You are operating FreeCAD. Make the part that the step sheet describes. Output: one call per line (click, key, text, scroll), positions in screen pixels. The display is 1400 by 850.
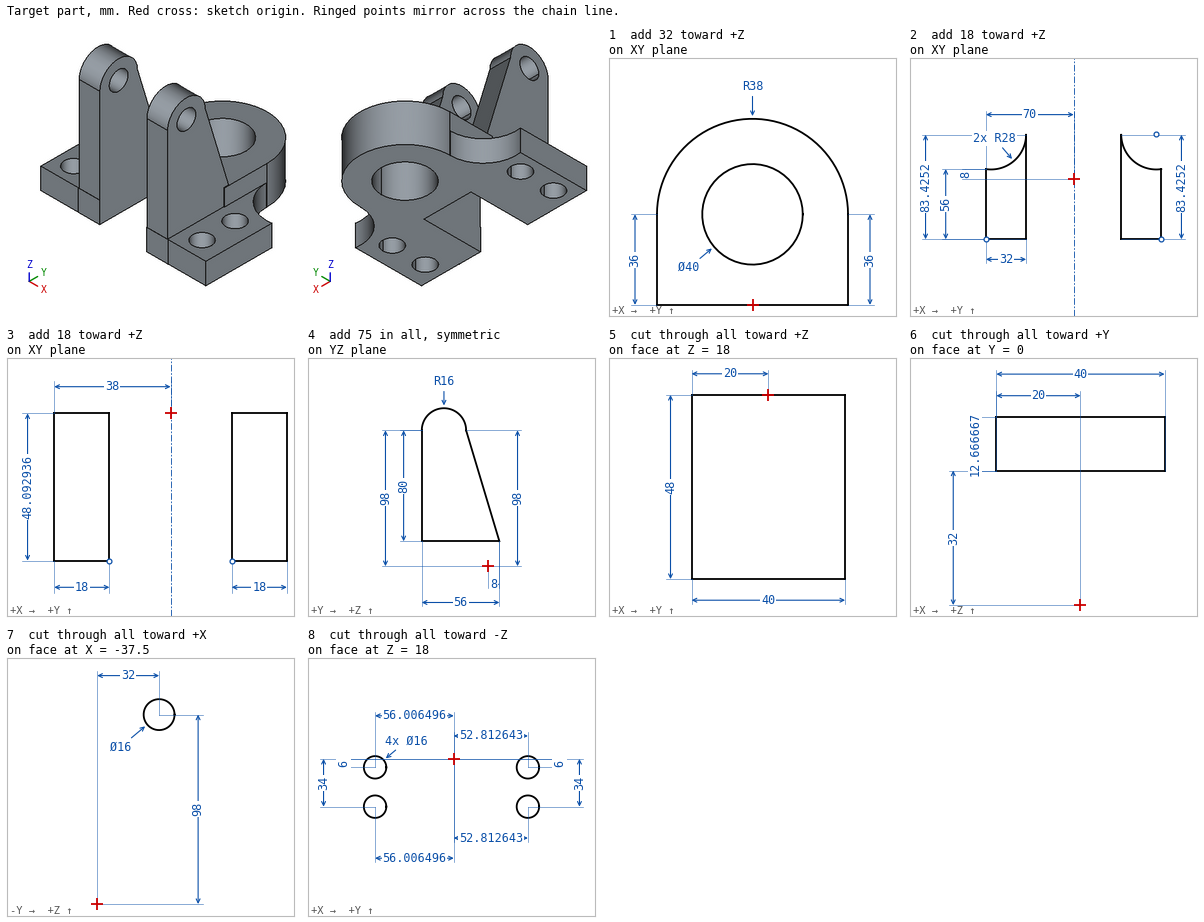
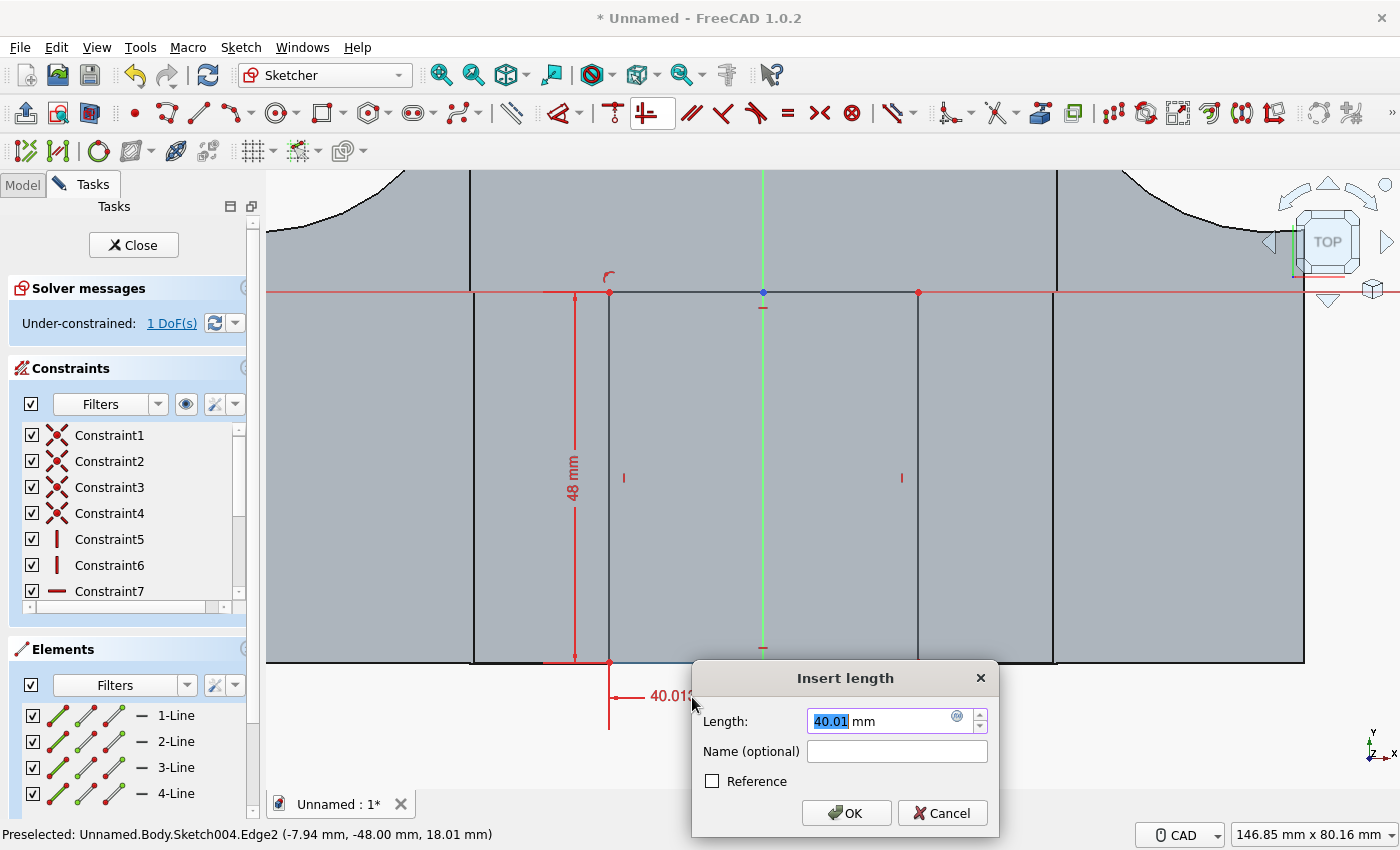
text(40)
key(Return)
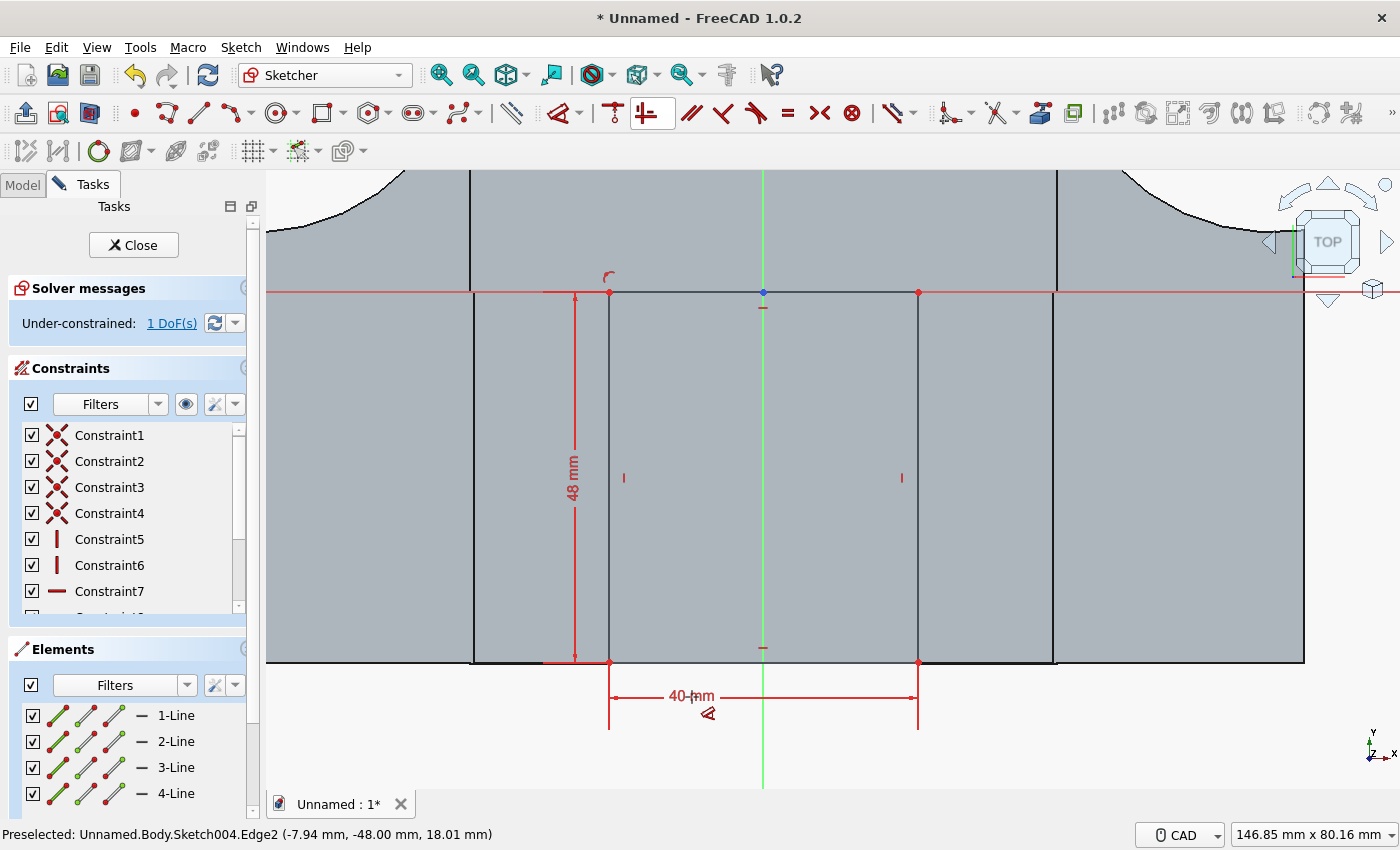
click(609, 292)
click(686, 258)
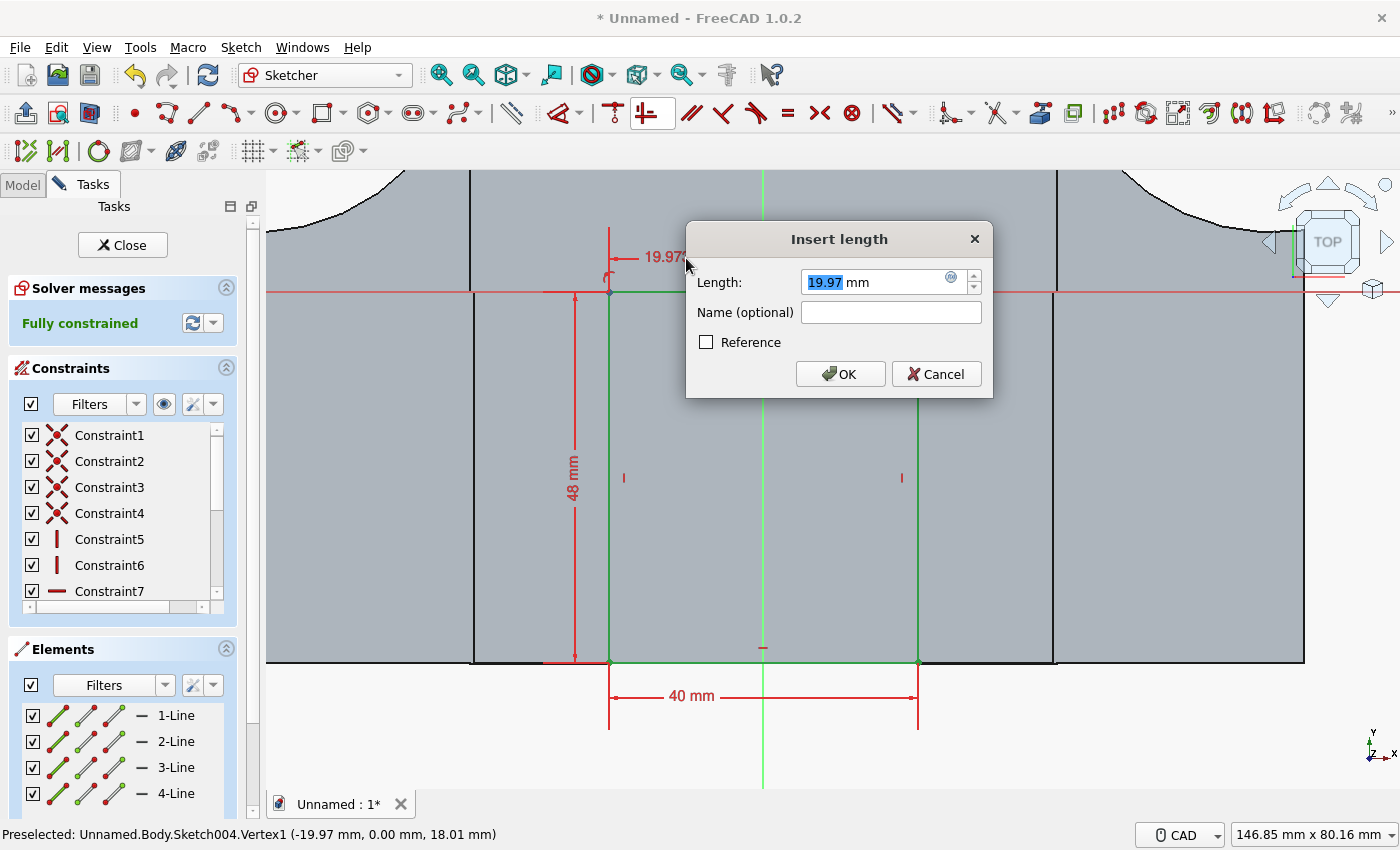
text(20)
key(Return)
key(Escape)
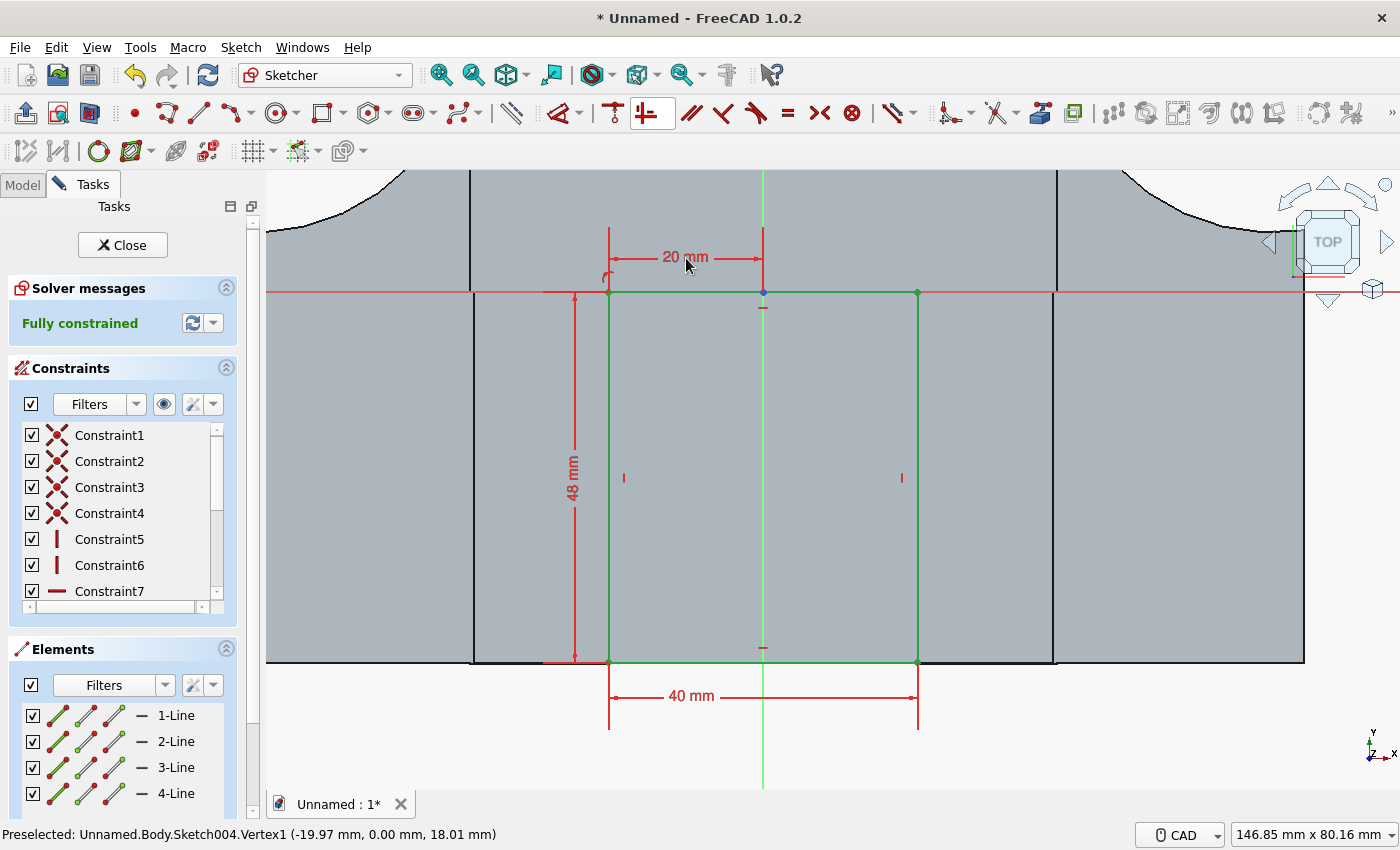
click(123, 245)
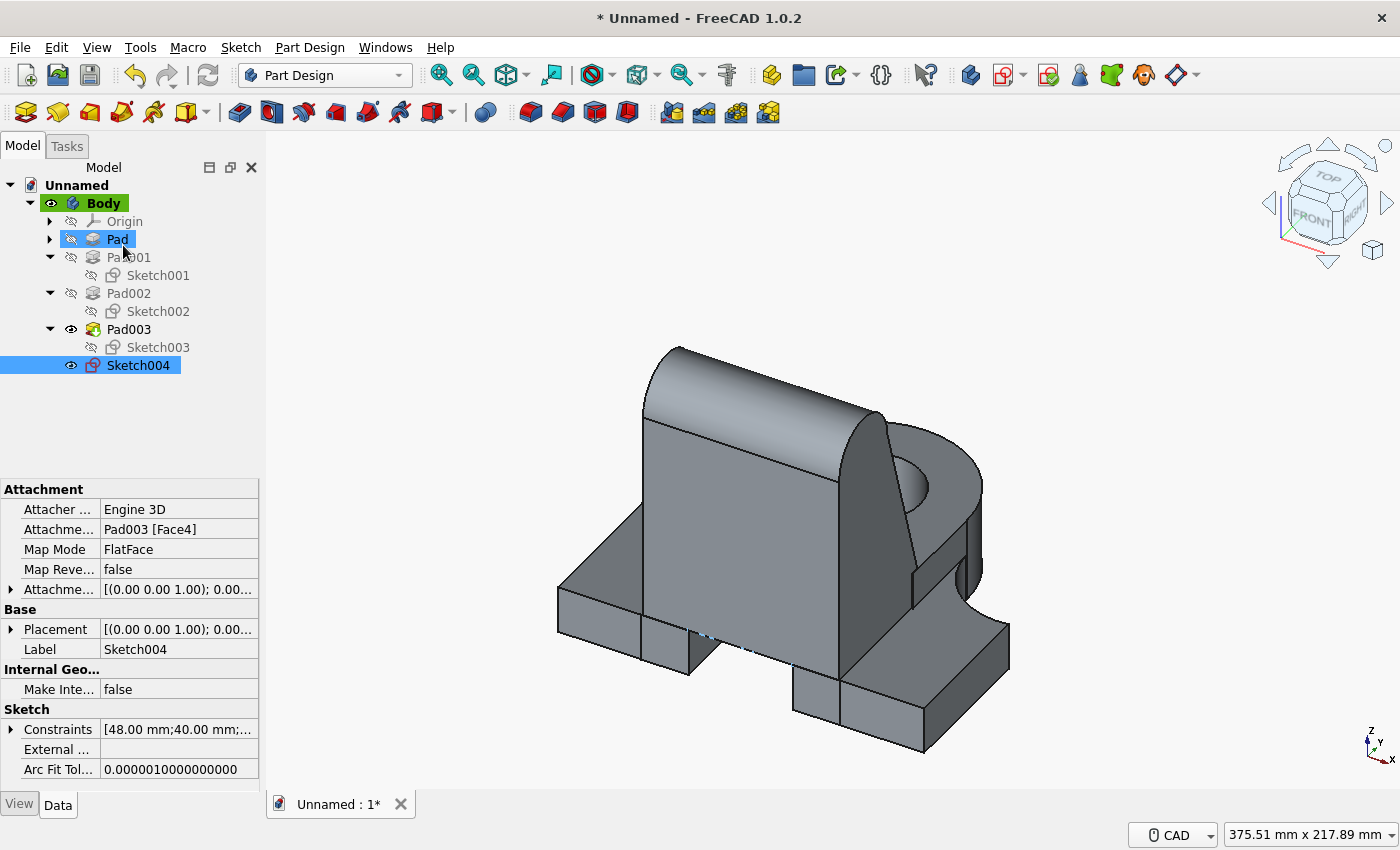
click(240, 112)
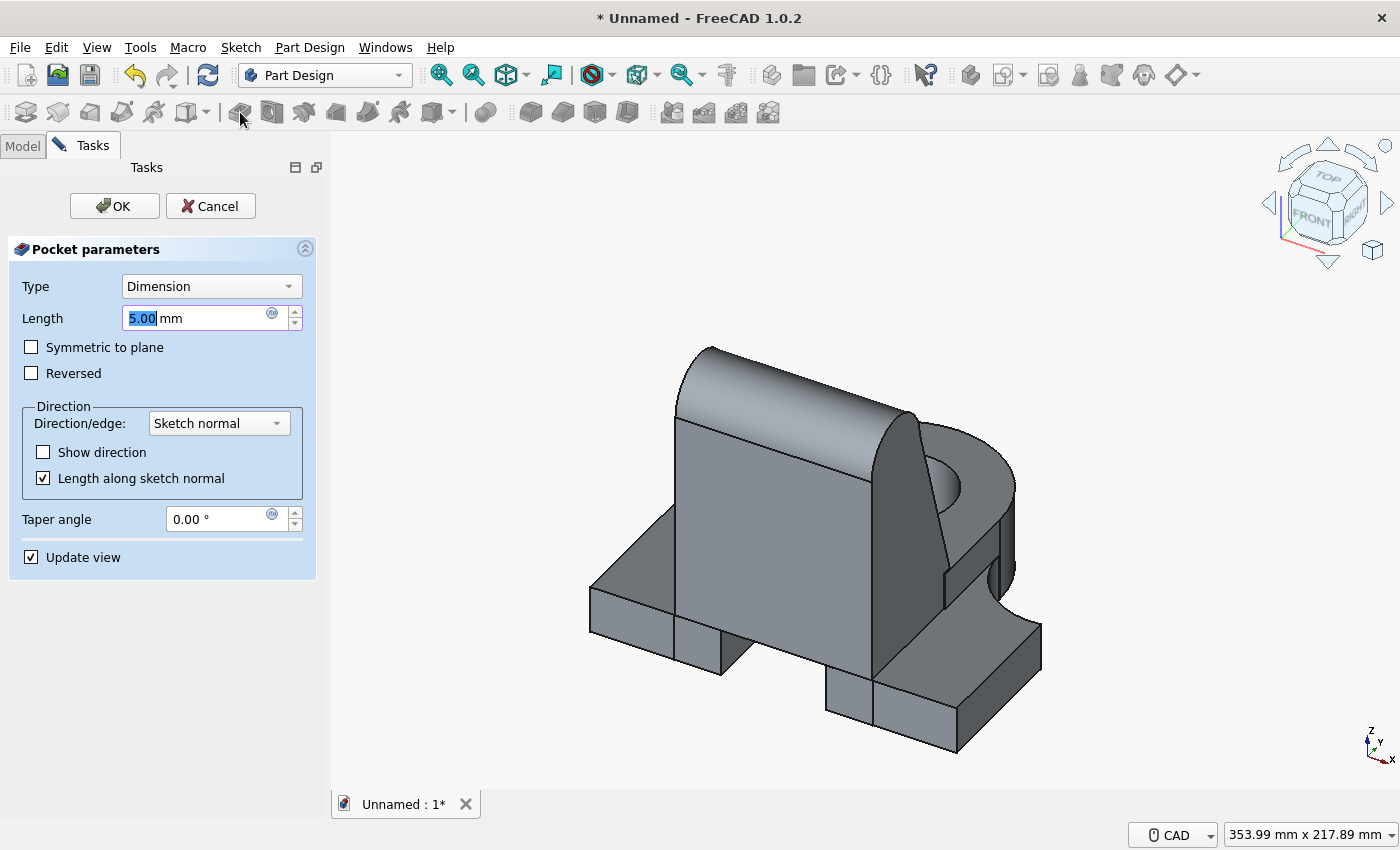
click(212, 286)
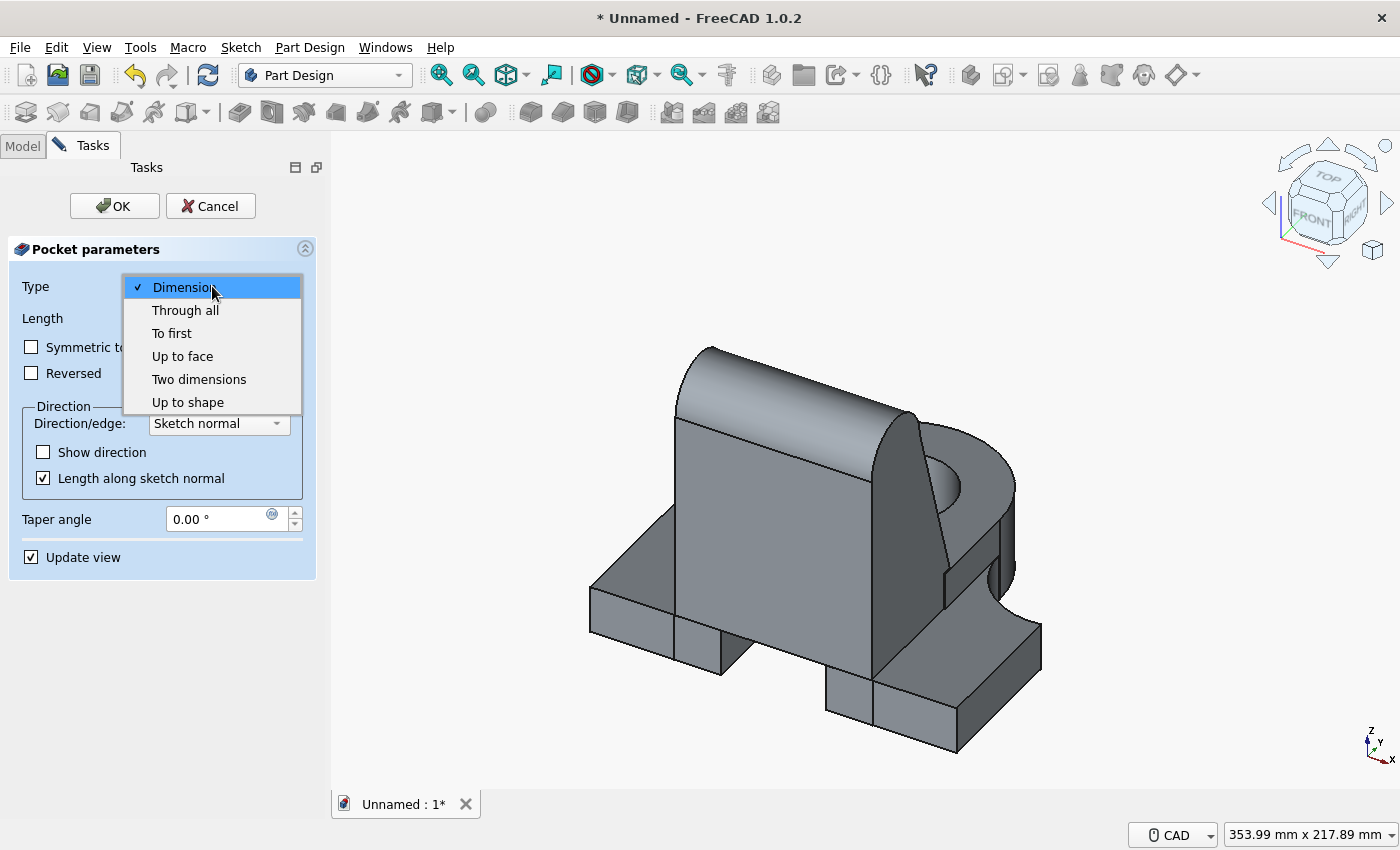
click(212, 310)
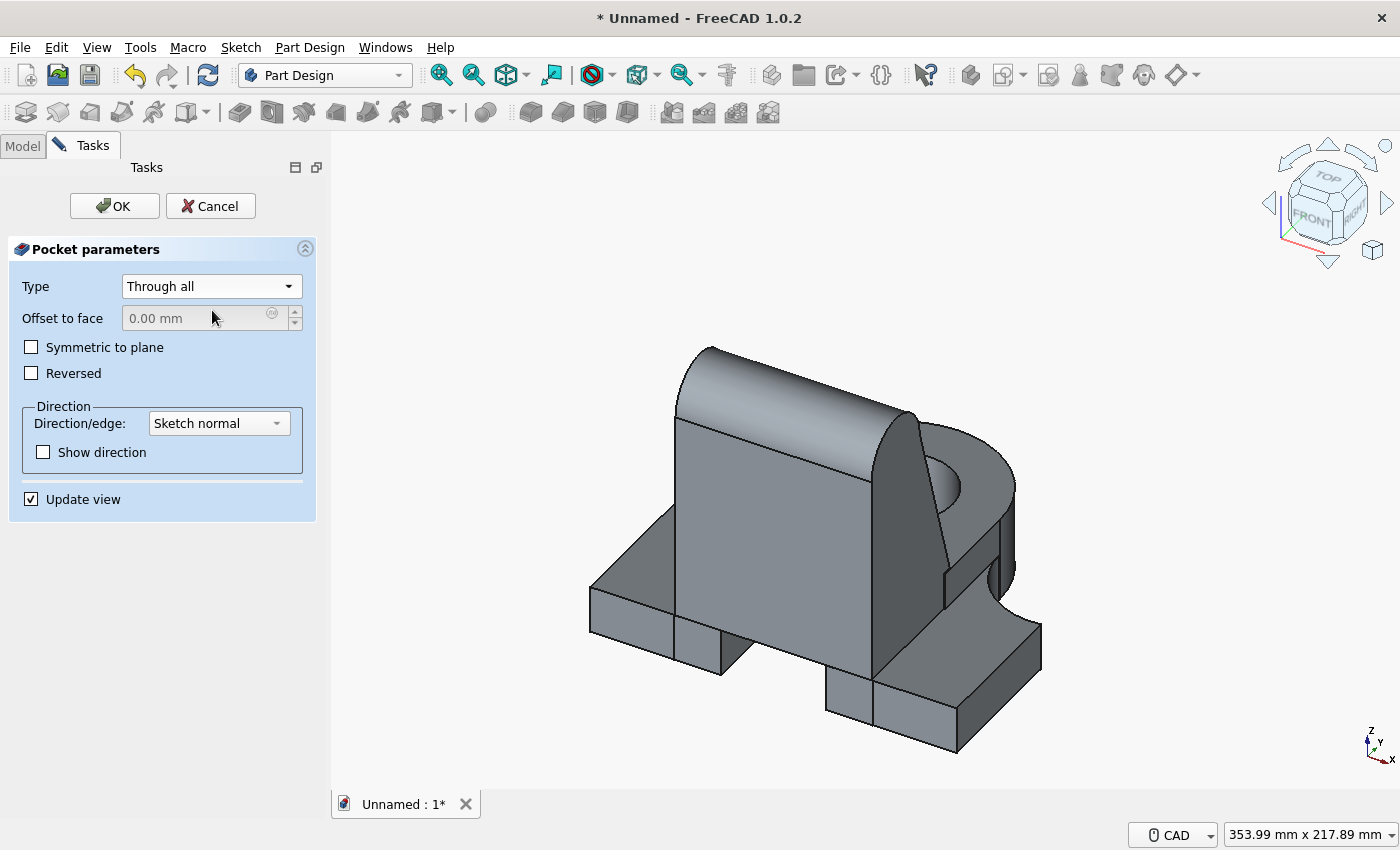
click(30, 373)